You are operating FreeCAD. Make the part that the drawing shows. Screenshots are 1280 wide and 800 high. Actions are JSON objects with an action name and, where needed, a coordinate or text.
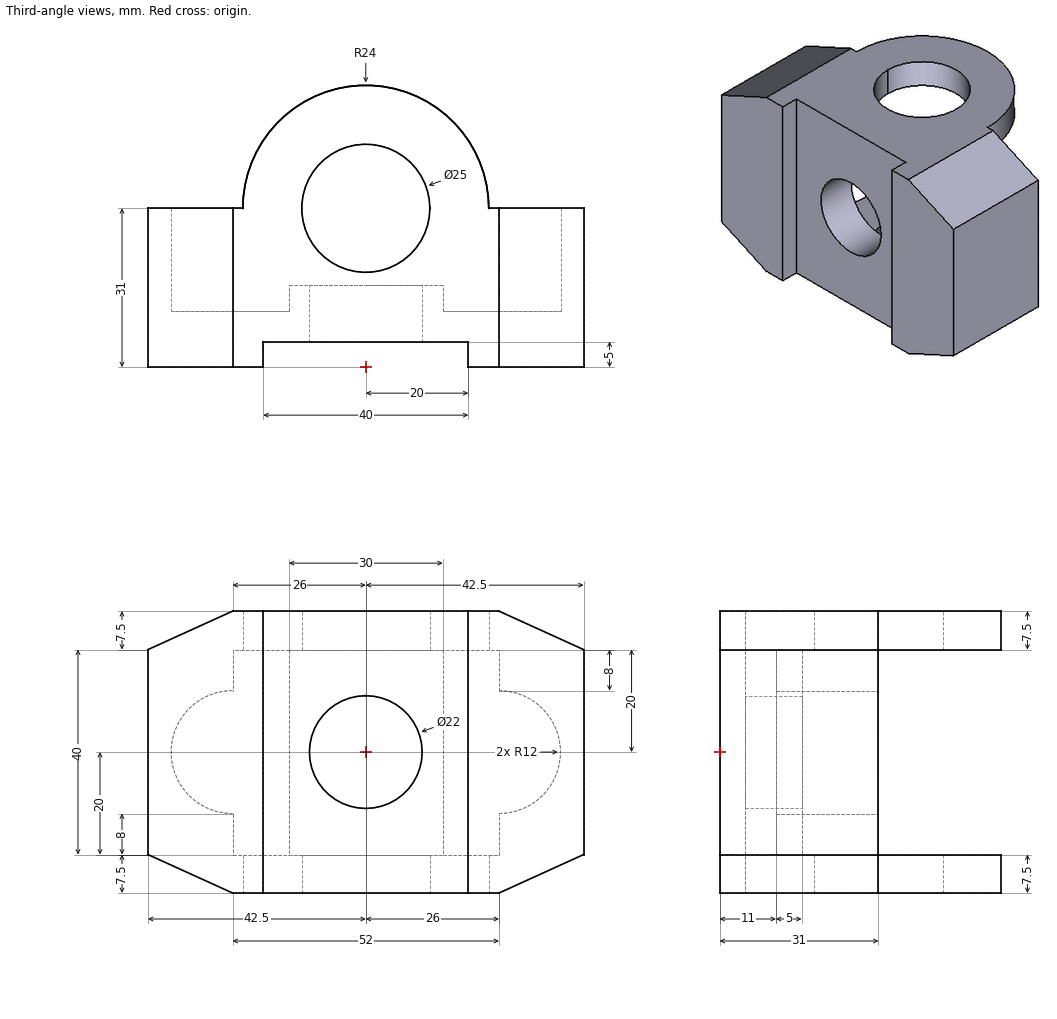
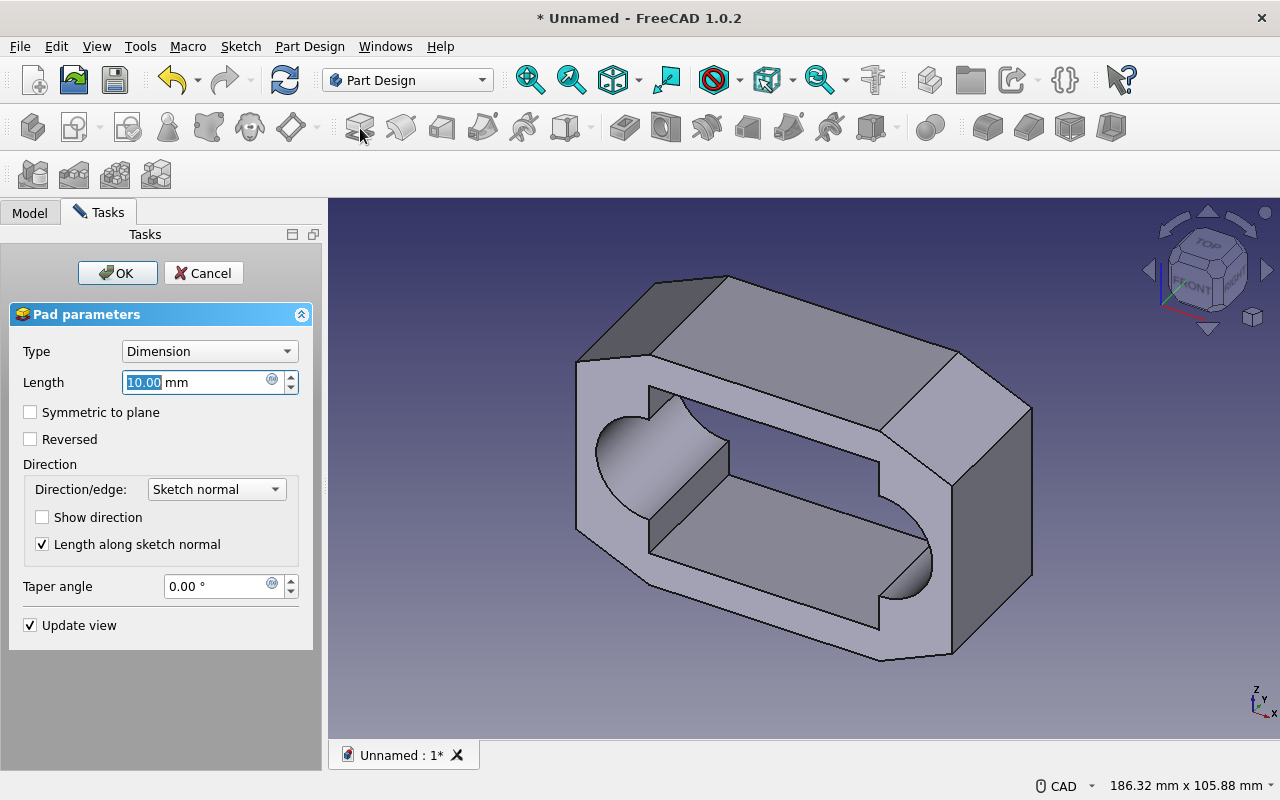
{"action": "type", "text": "7.5"}
{"action": "key", "text": "Tab"}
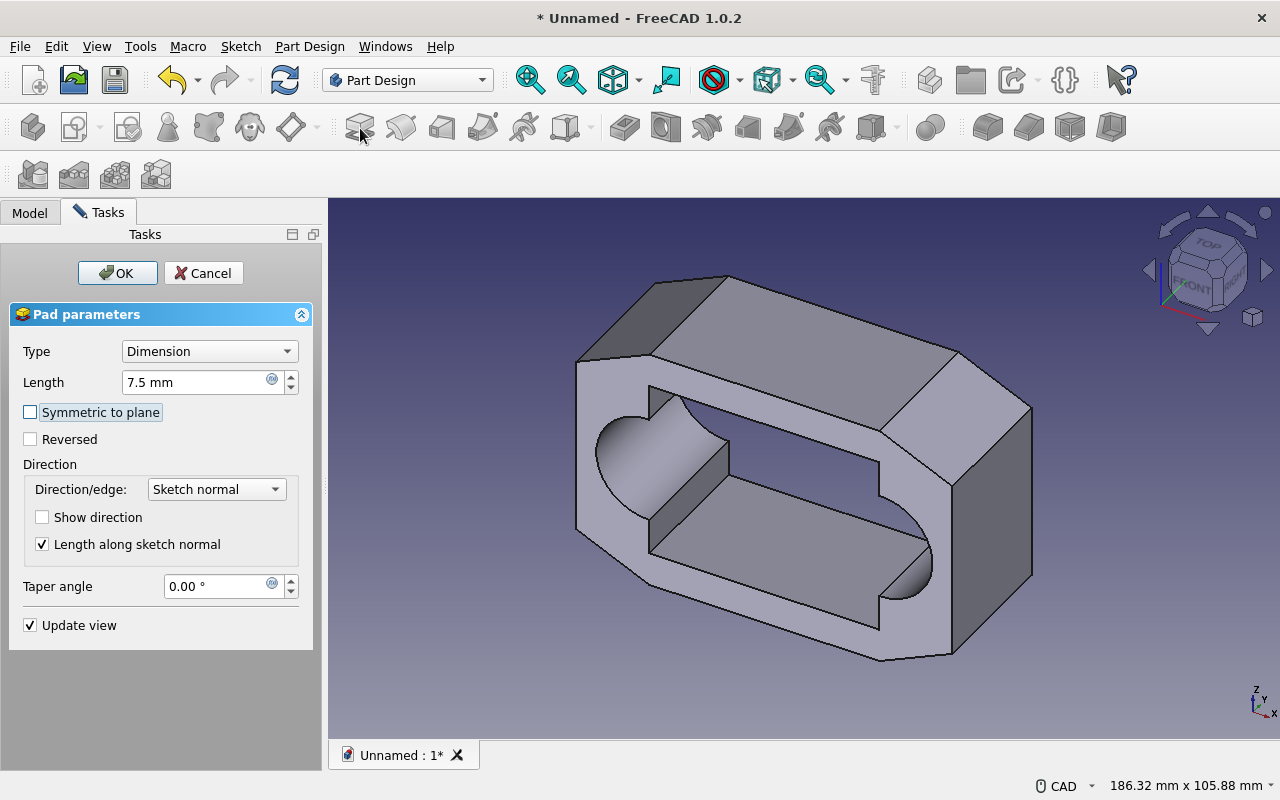
{"action": "left_click", "coordinate": [31, 439]}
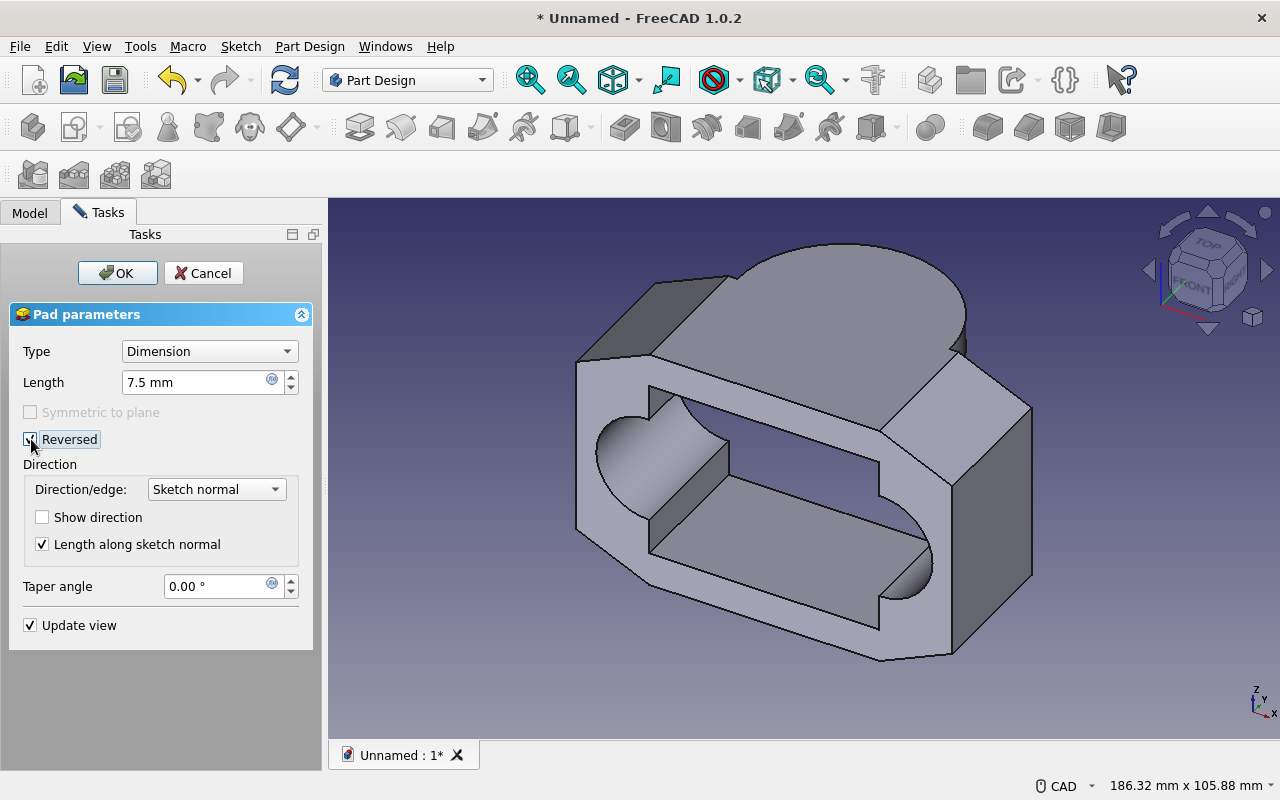
{"action": "left_click", "coordinate": [118, 273]}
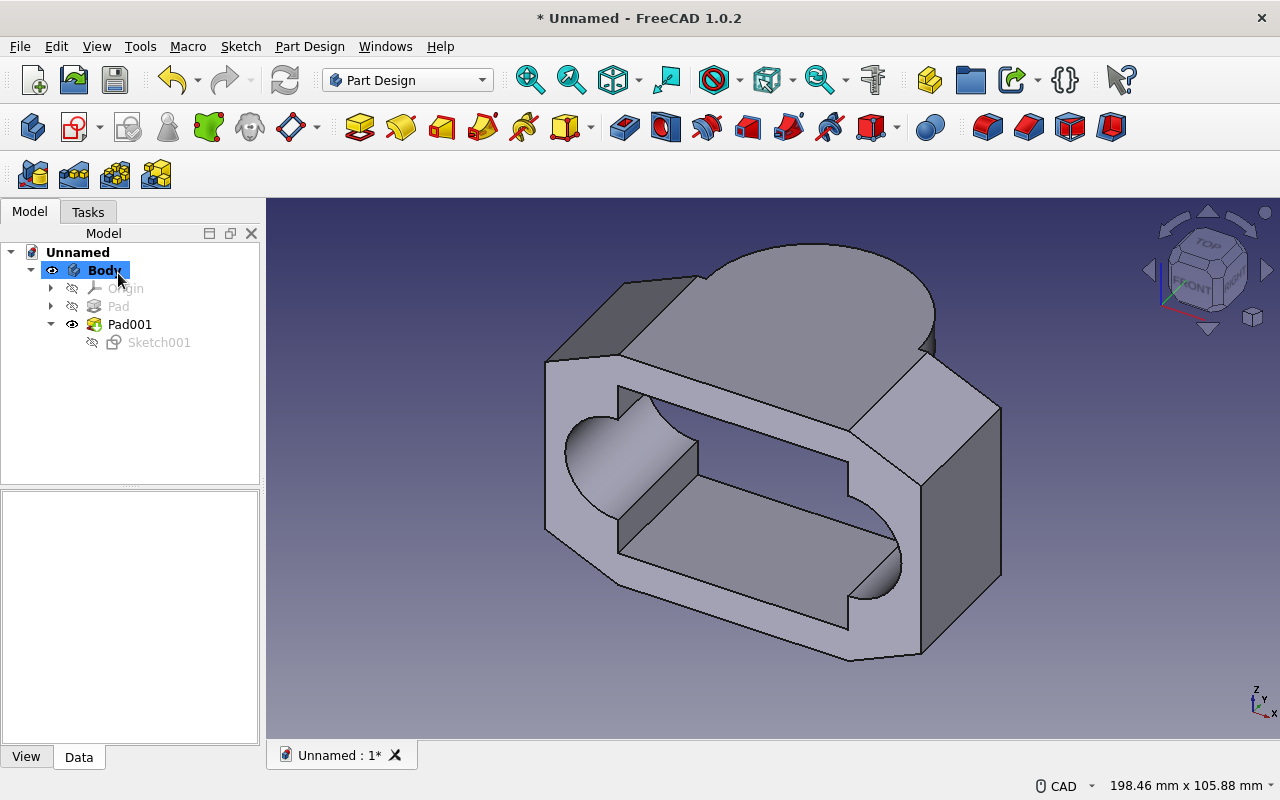
{"action": "left_click", "coordinate": [531, 80]}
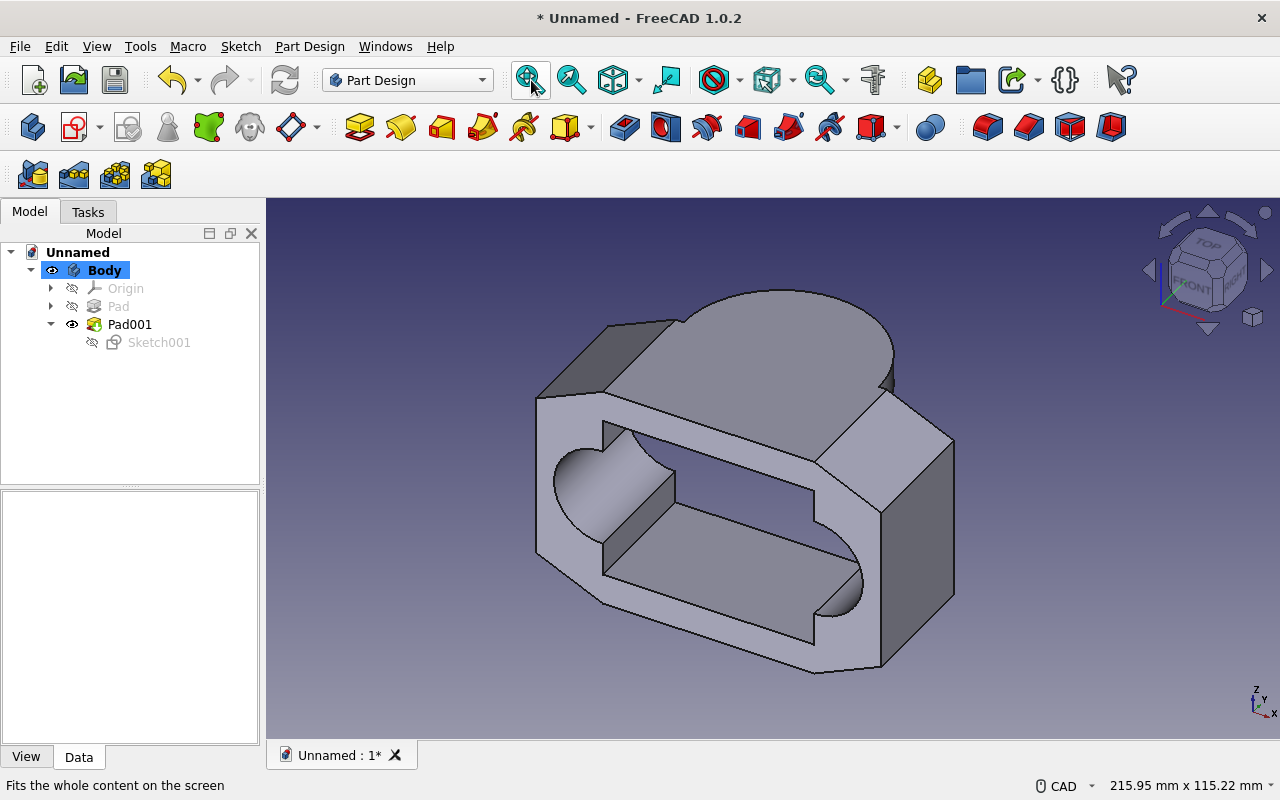
{"action": "left_click", "coordinate": [51, 288]}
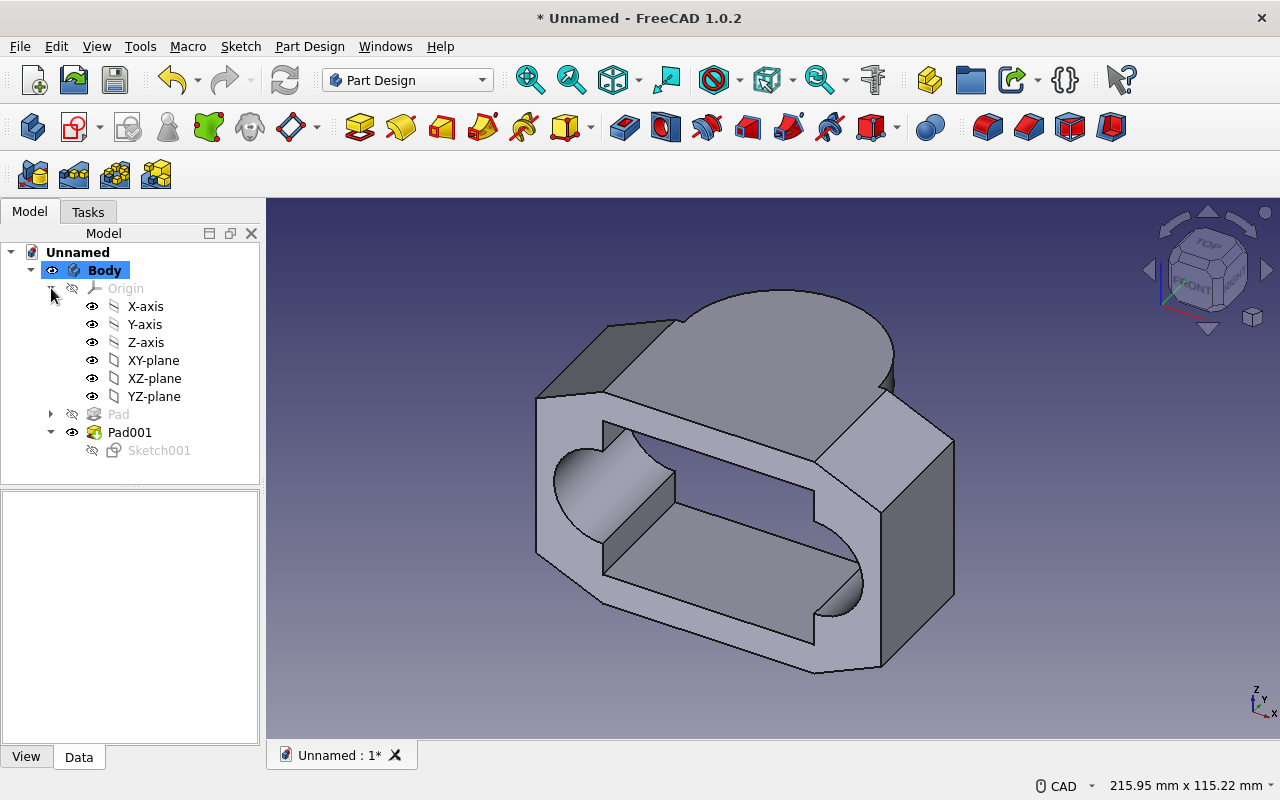
{"action": "left_click", "coordinate": [137, 360]}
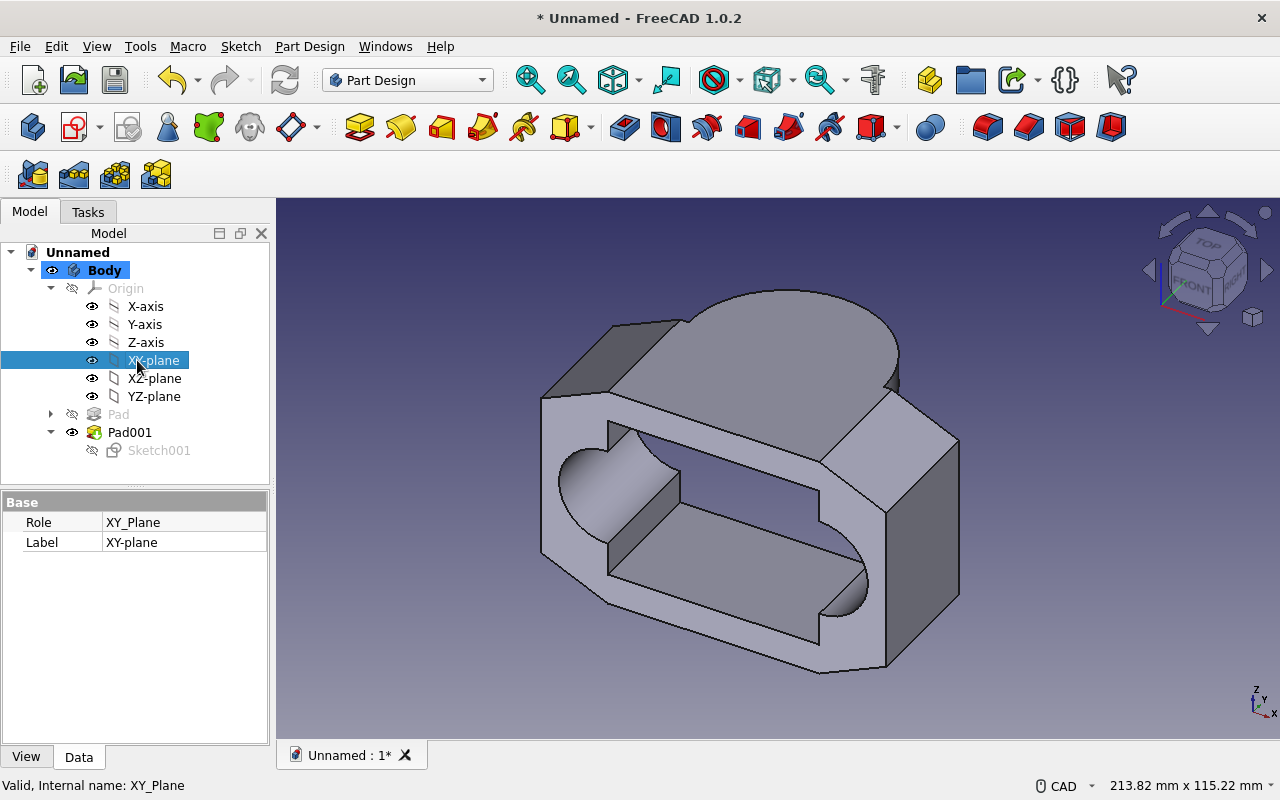
{"action": "left_click", "coordinate": [290, 128]}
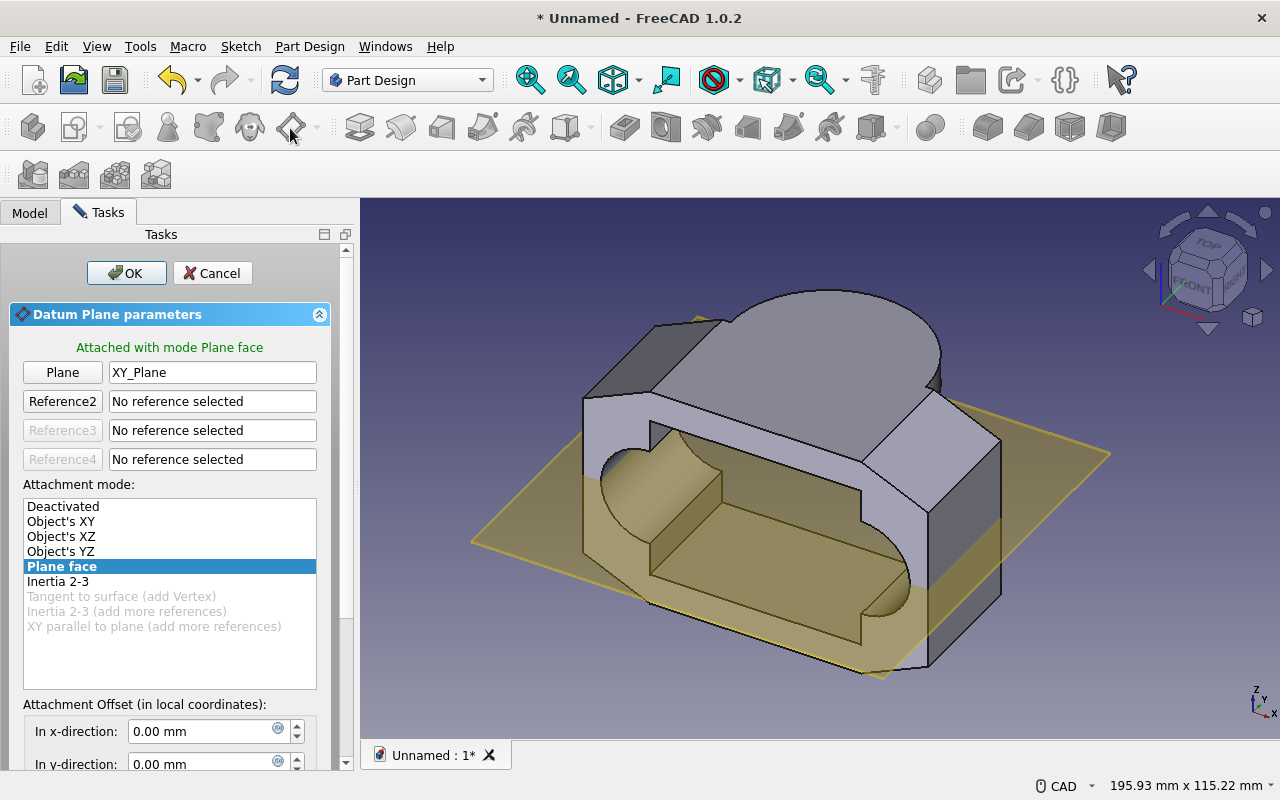
{"action": "scroll", "coordinate": [346, 507], "scroll_direction": "down", "scroll_amount": 2}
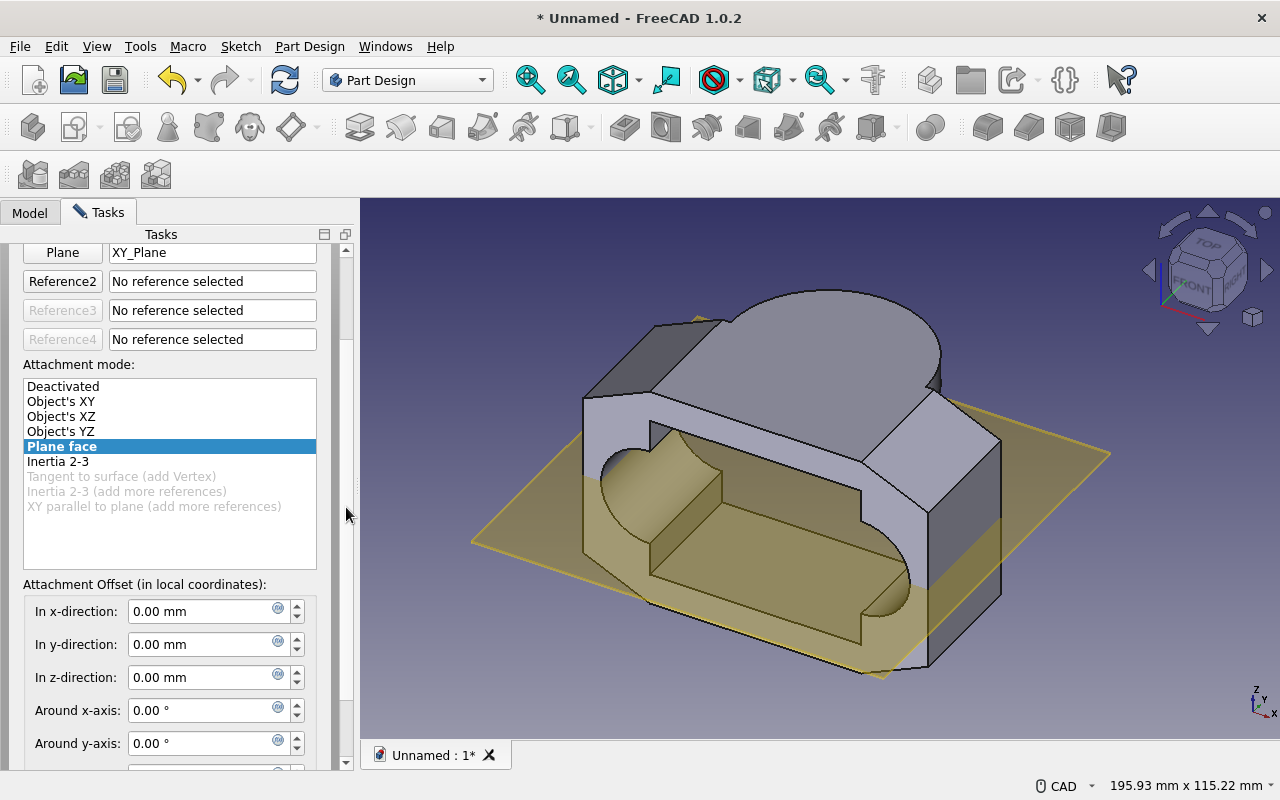
{"action": "triple_click", "coordinate": [210, 678]}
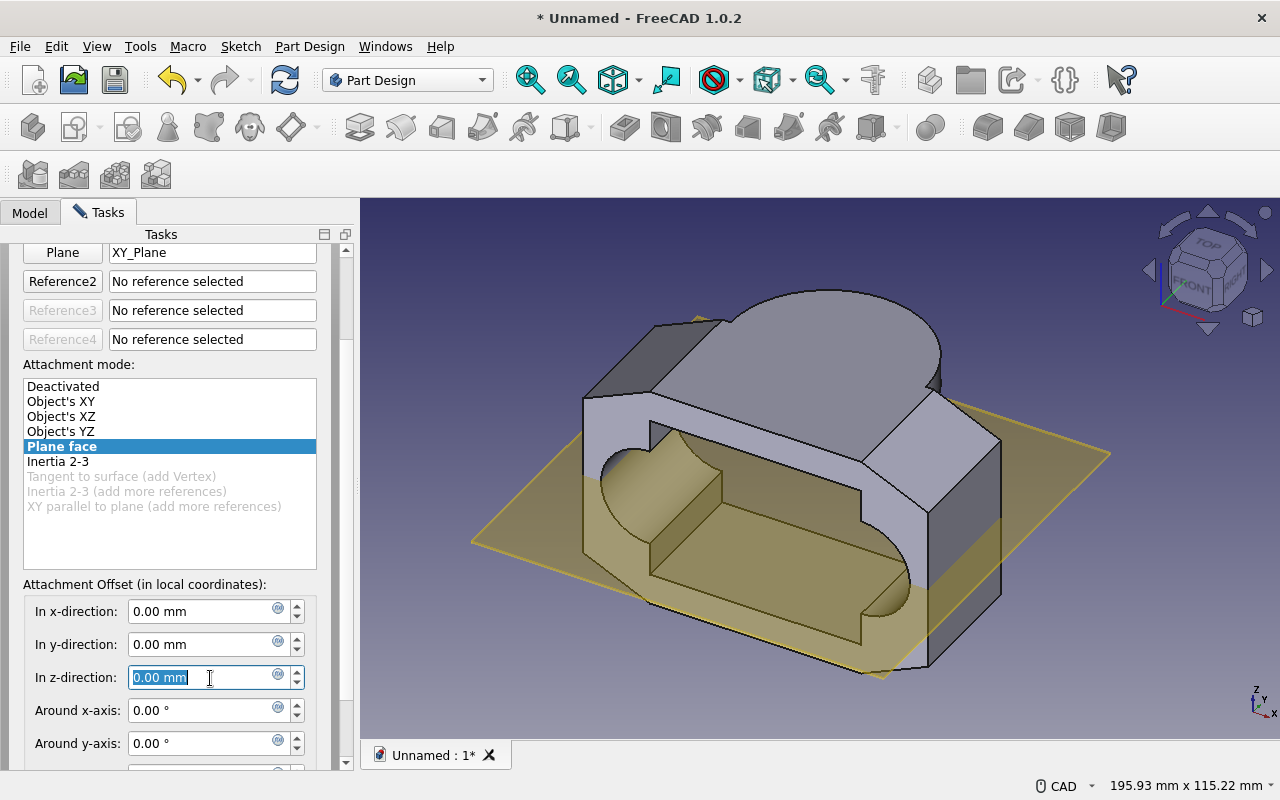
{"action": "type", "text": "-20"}
{"action": "key", "text": "Tab"}